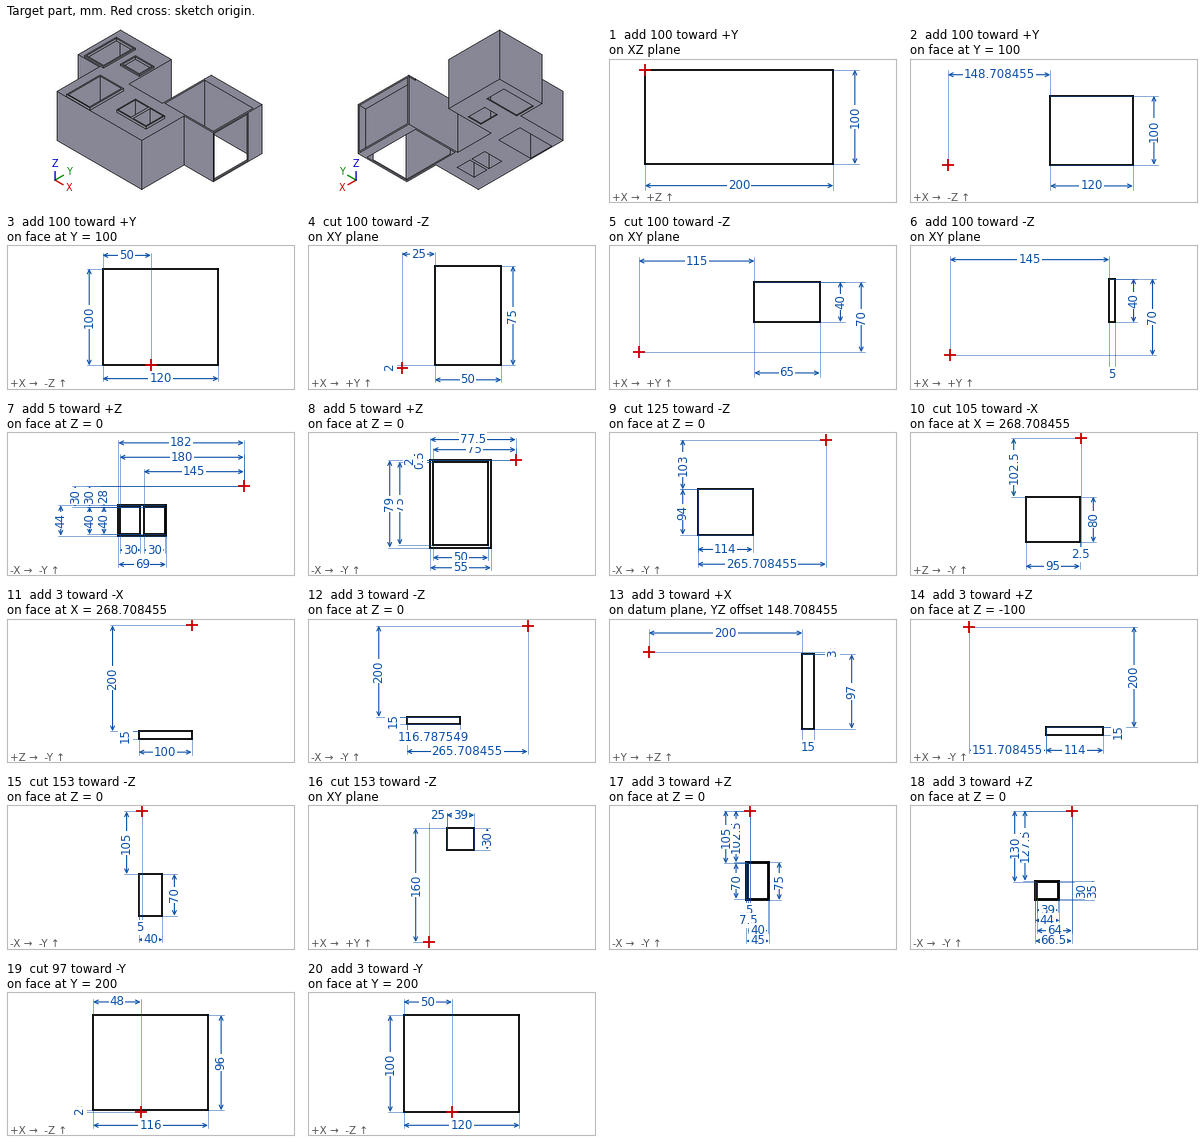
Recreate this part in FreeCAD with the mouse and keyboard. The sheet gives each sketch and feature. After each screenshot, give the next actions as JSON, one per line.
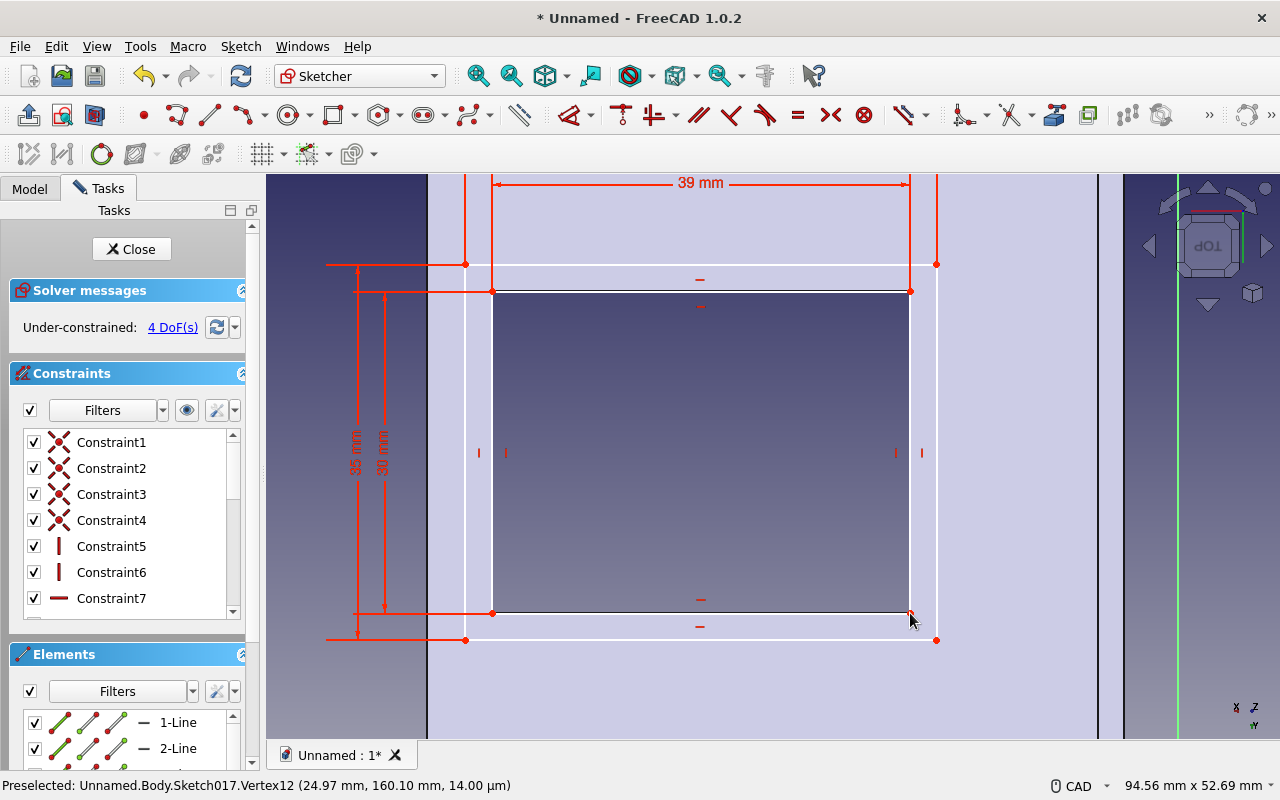
{"action": "left_click", "coordinate": [568, 116]}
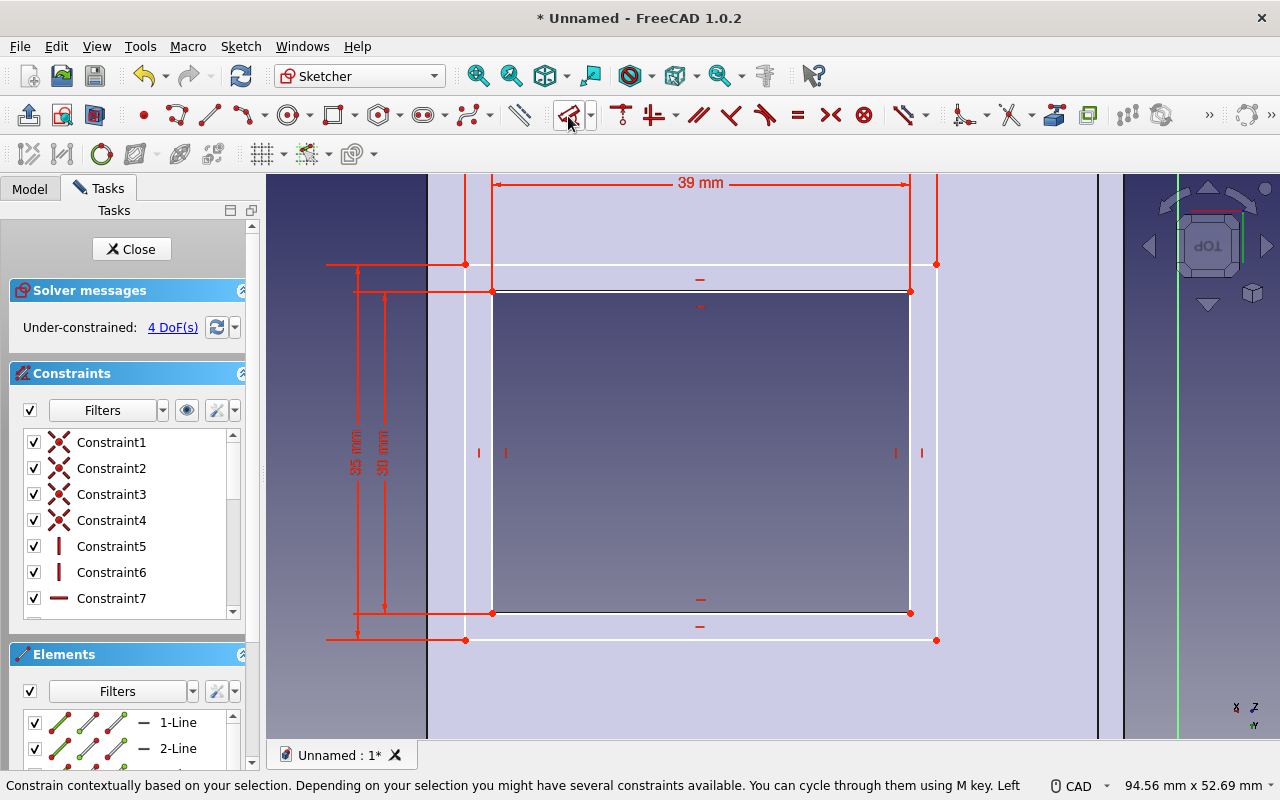
{"action": "left_click", "coordinate": [492, 292]}
{"action": "left_click", "coordinate": [804, 326]}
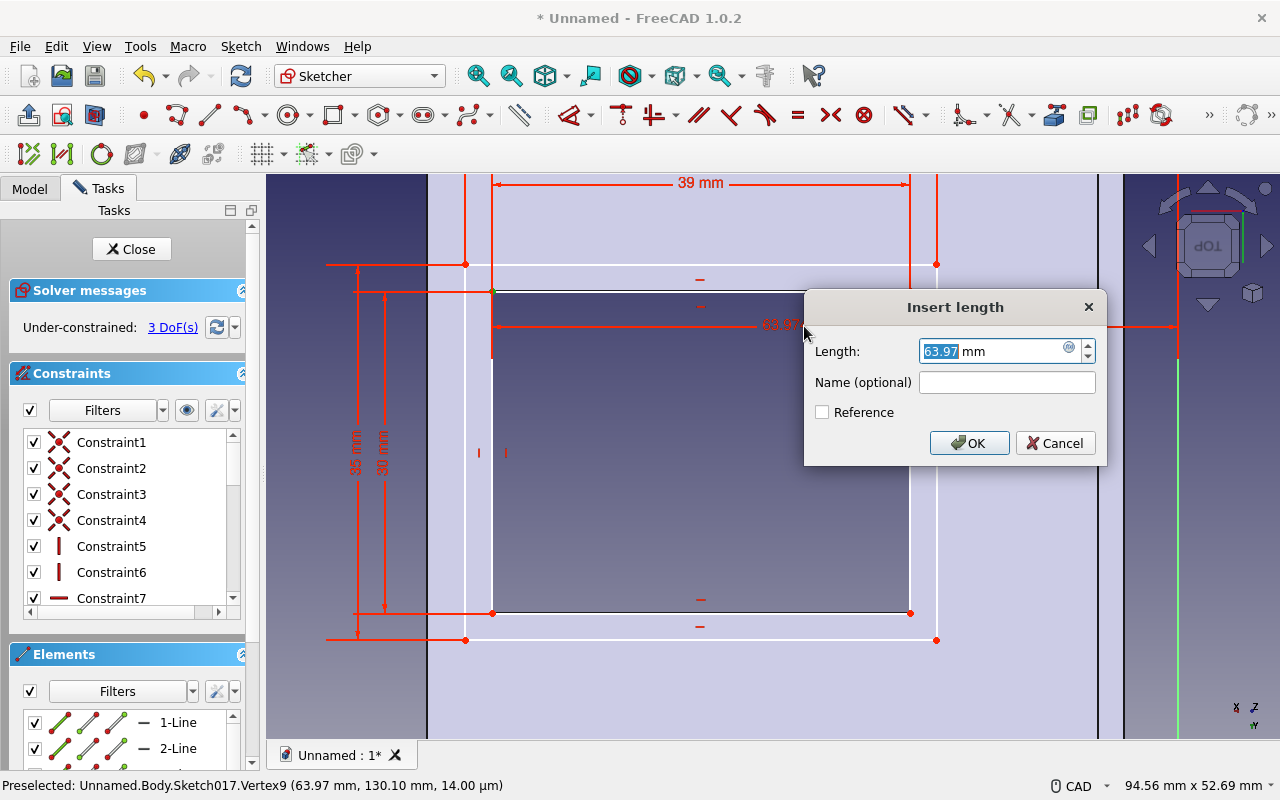
{"action": "type", "text": "64"}
{"action": "key", "text": "Return"}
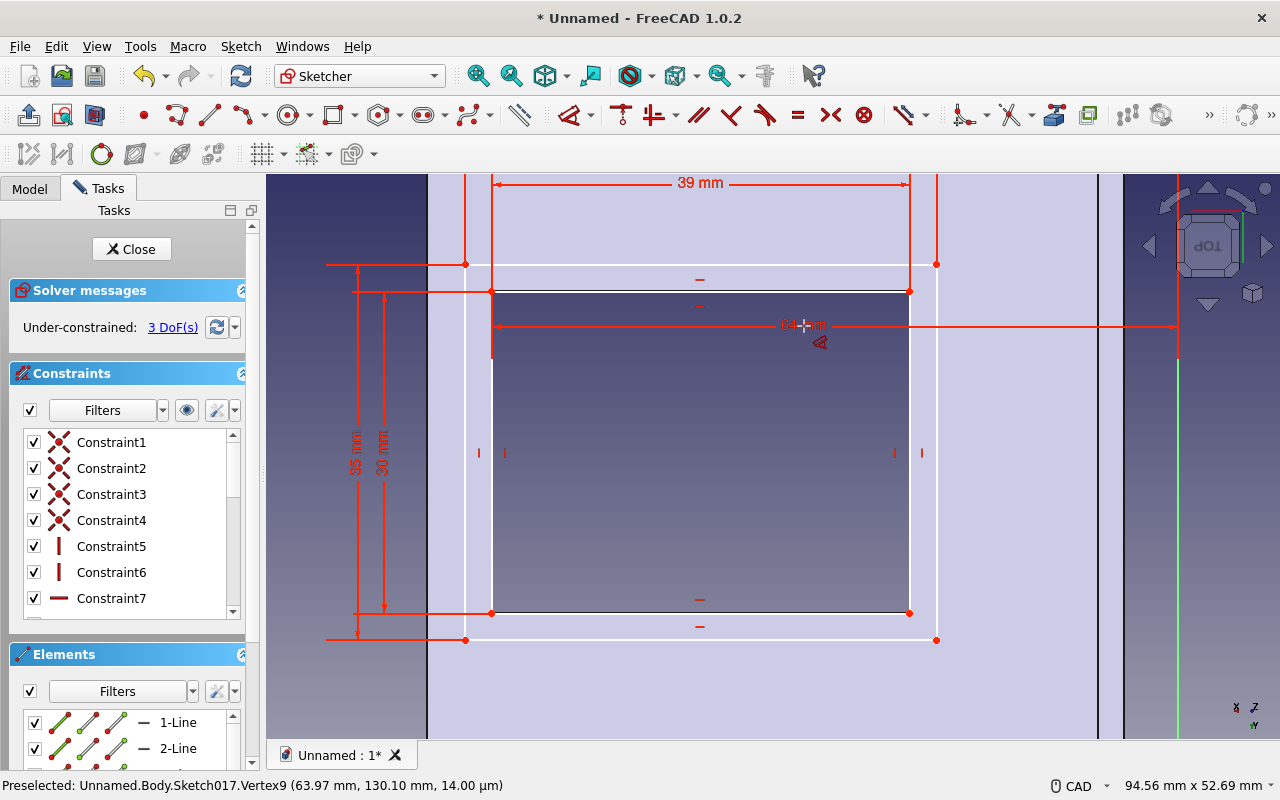
{"action": "left_click", "coordinate": [492, 292]}
{"action": "left_click", "coordinate": [458, 247]}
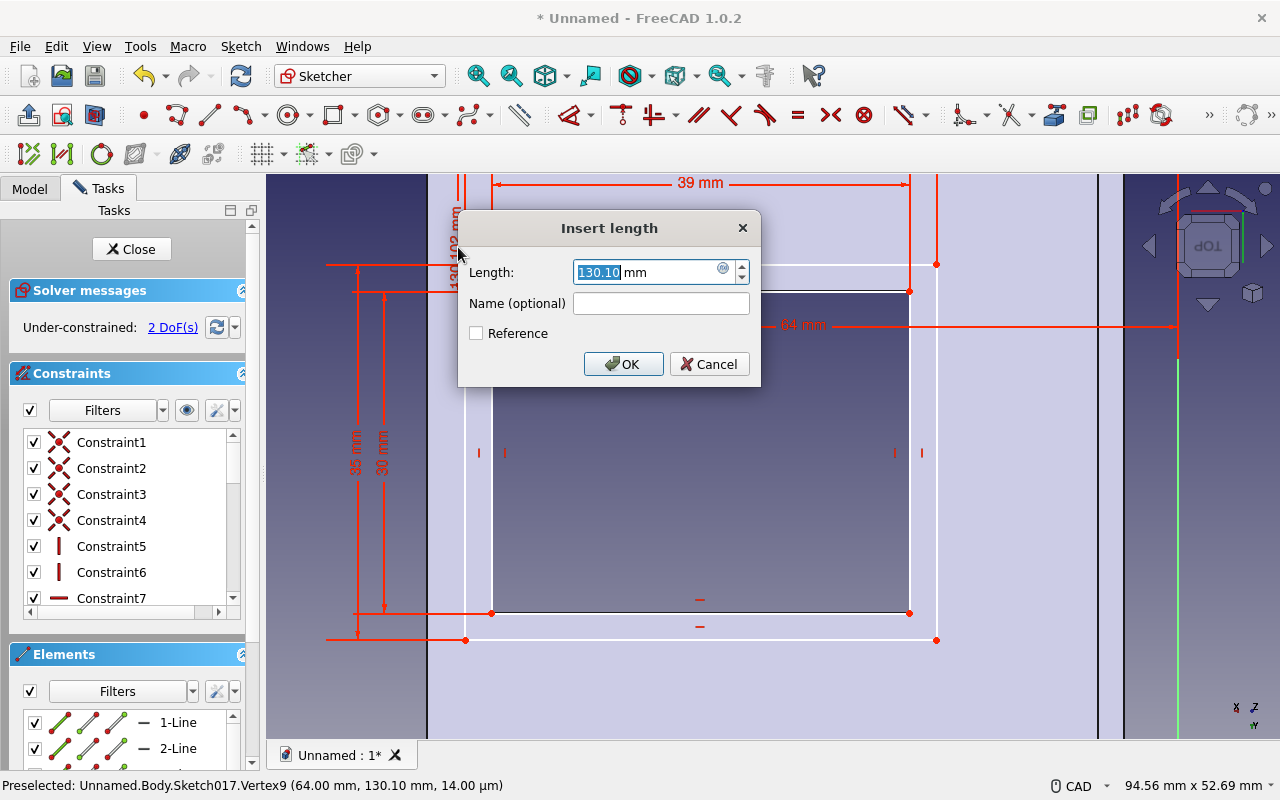
{"action": "type", "text": "130"}
{"action": "key", "text": "Return"}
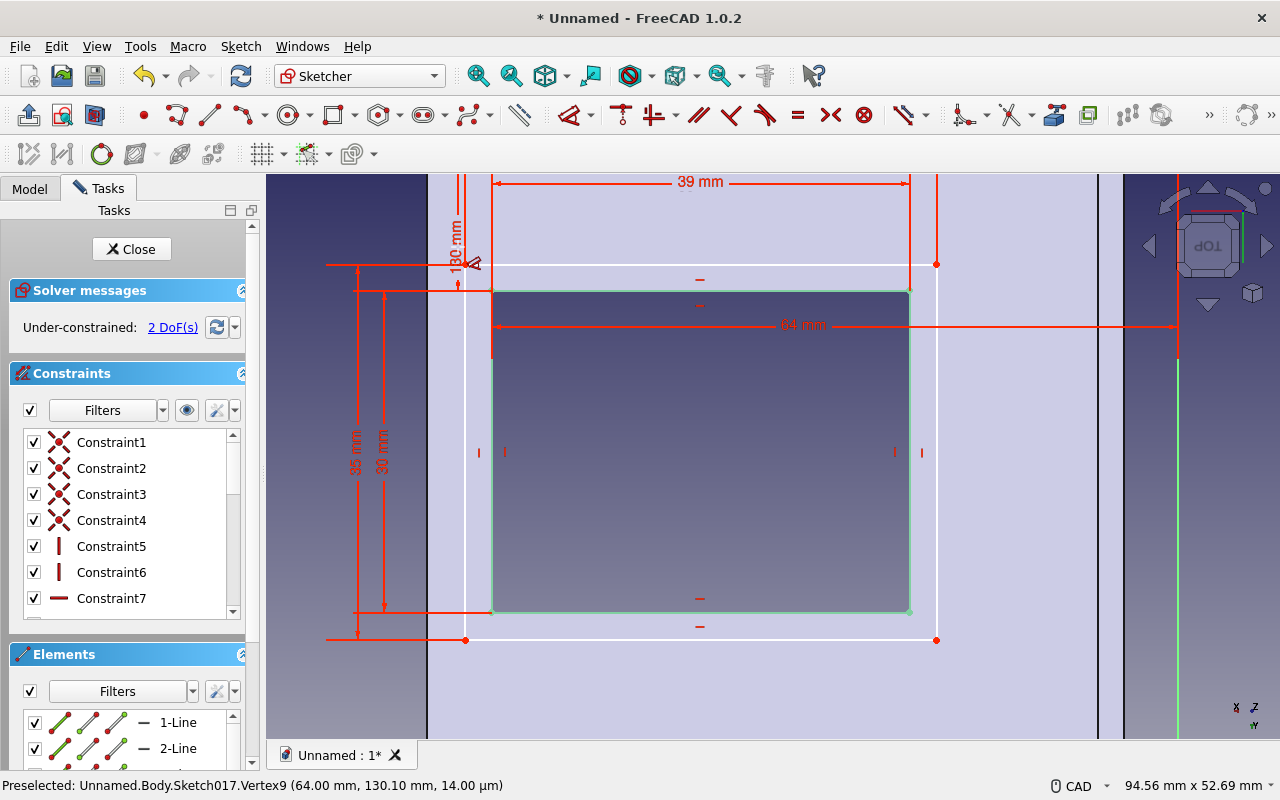
{"action": "left_click", "coordinate": [465, 265]}
{"action": "left_click", "coordinate": [1017, 299]}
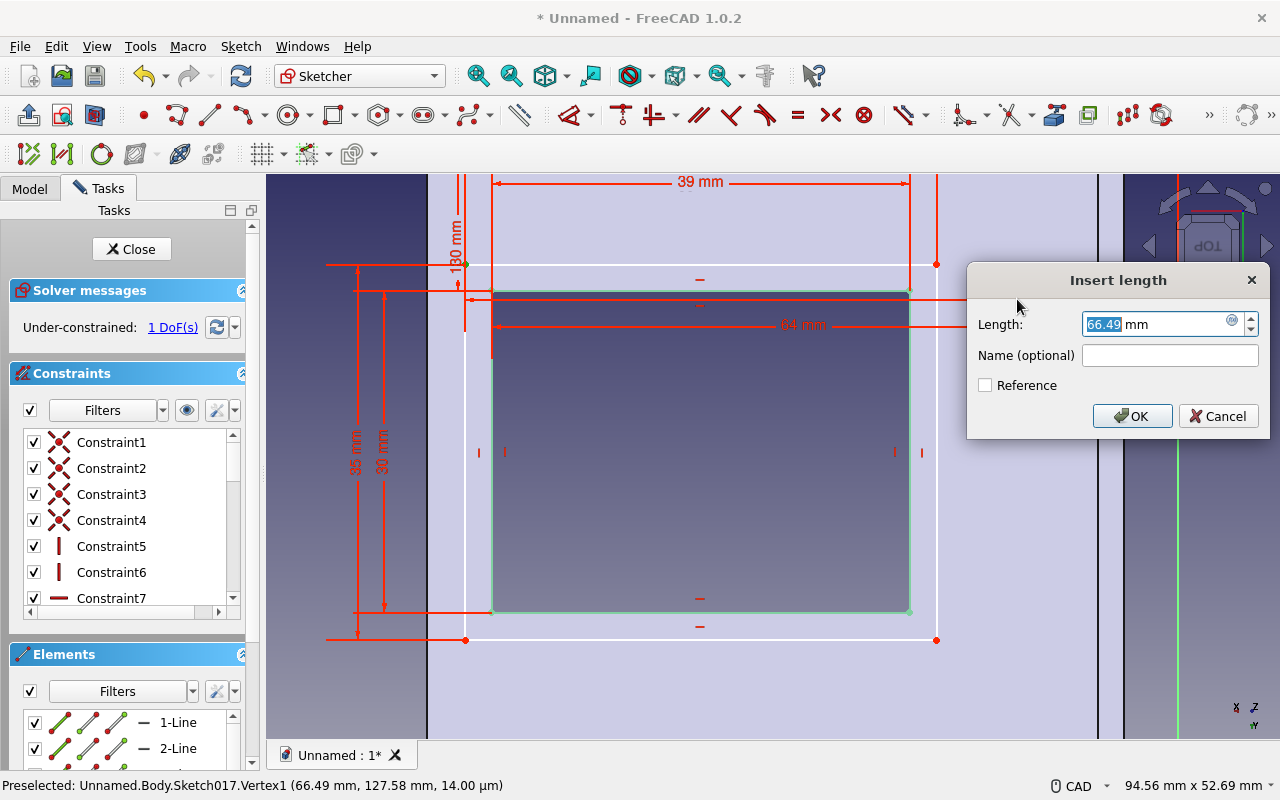
{"action": "type", "text": "66.5"}
{"action": "key", "text": "Return"}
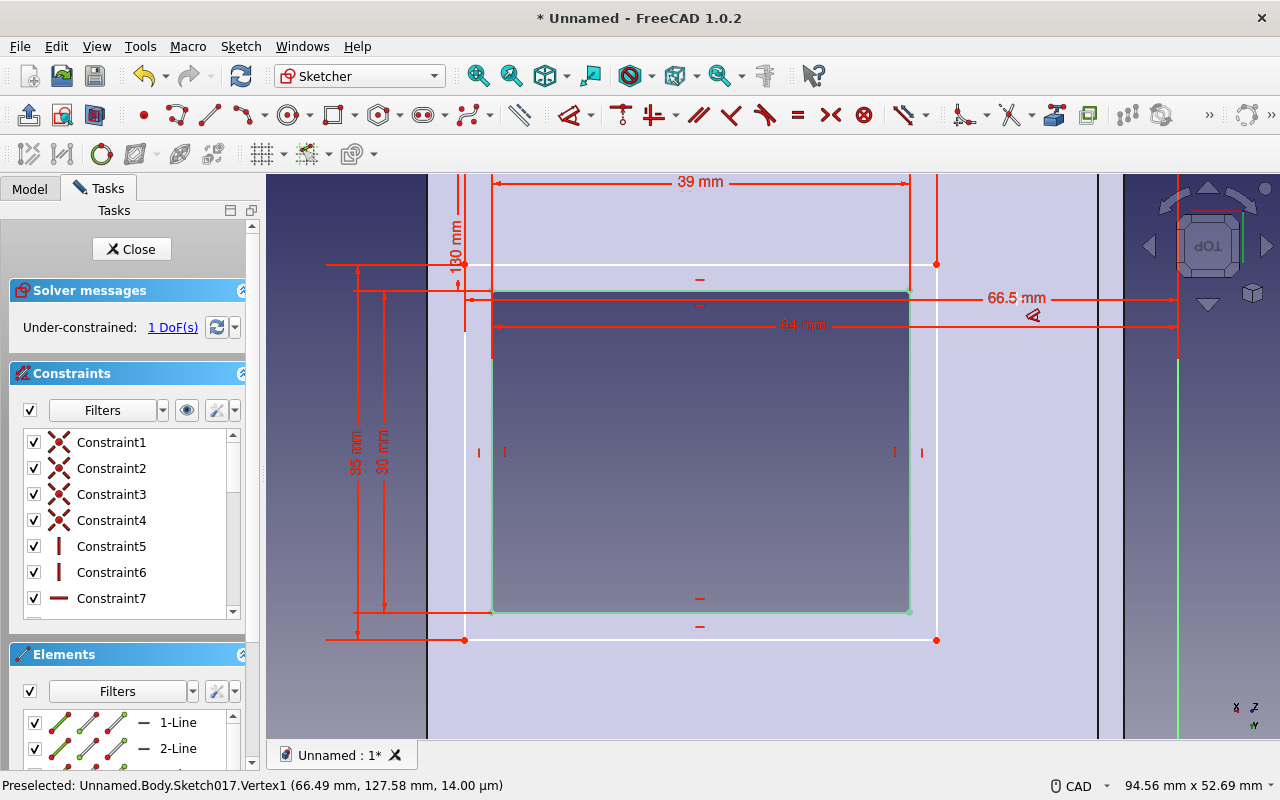
{"action": "left_click", "coordinate": [465, 265]}
{"action": "left_click", "coordinate": [431, 219]}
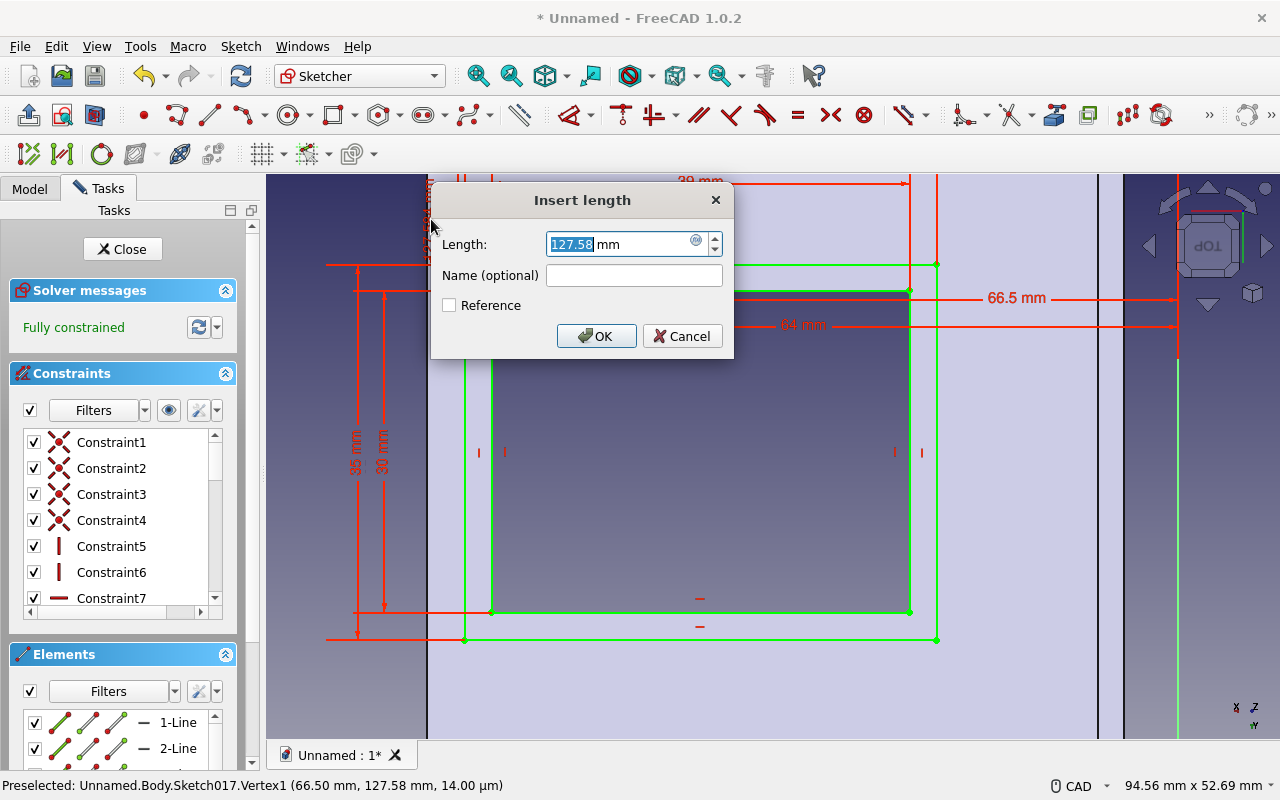
{"action": "type", "text": "127.5"}
{"action": "key", "text": "Return"}
{"action": "key", "text": "Escape"}